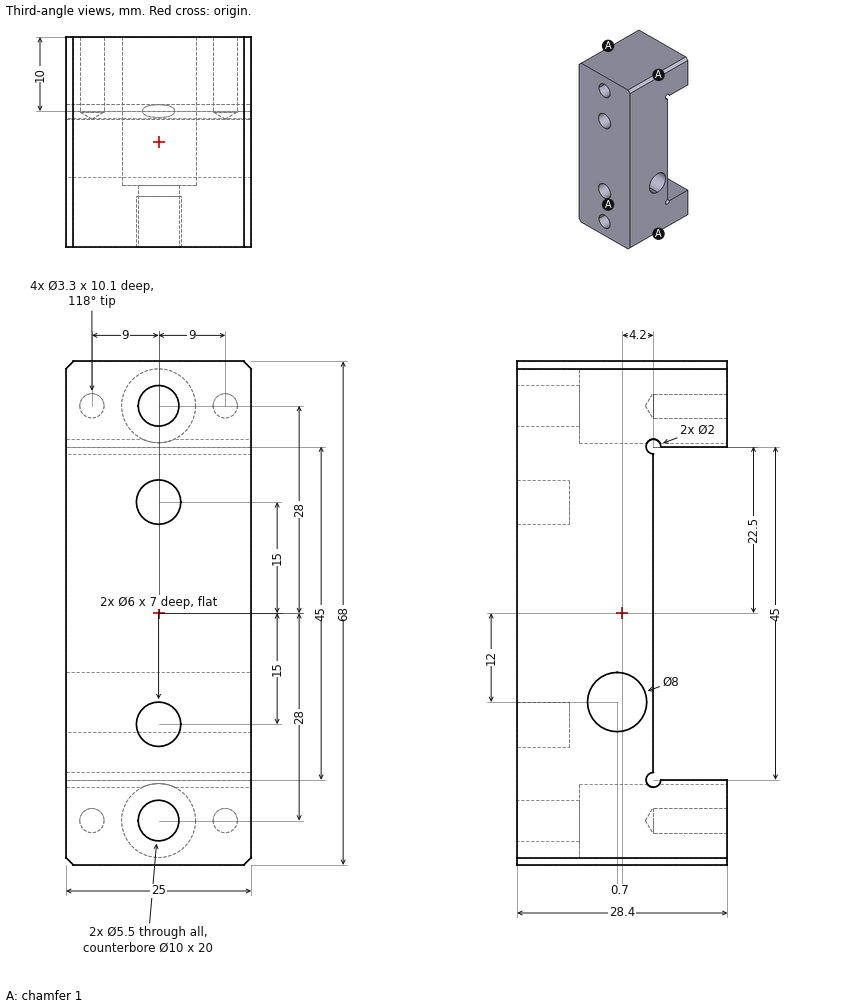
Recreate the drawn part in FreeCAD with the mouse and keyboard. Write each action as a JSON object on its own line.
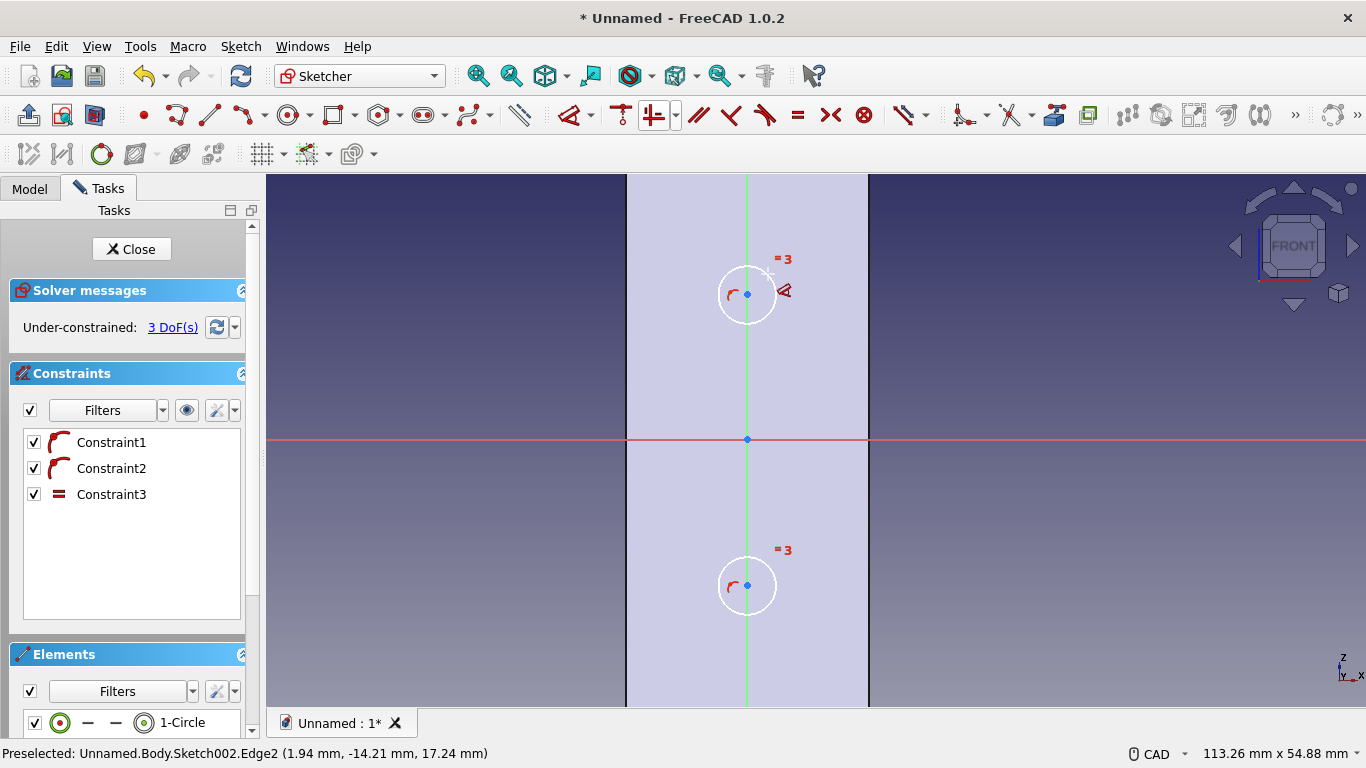
{"action": "left_click", "coordinate": [768, 566]}
{"action": "left_click", "coordinate": [791, 544]}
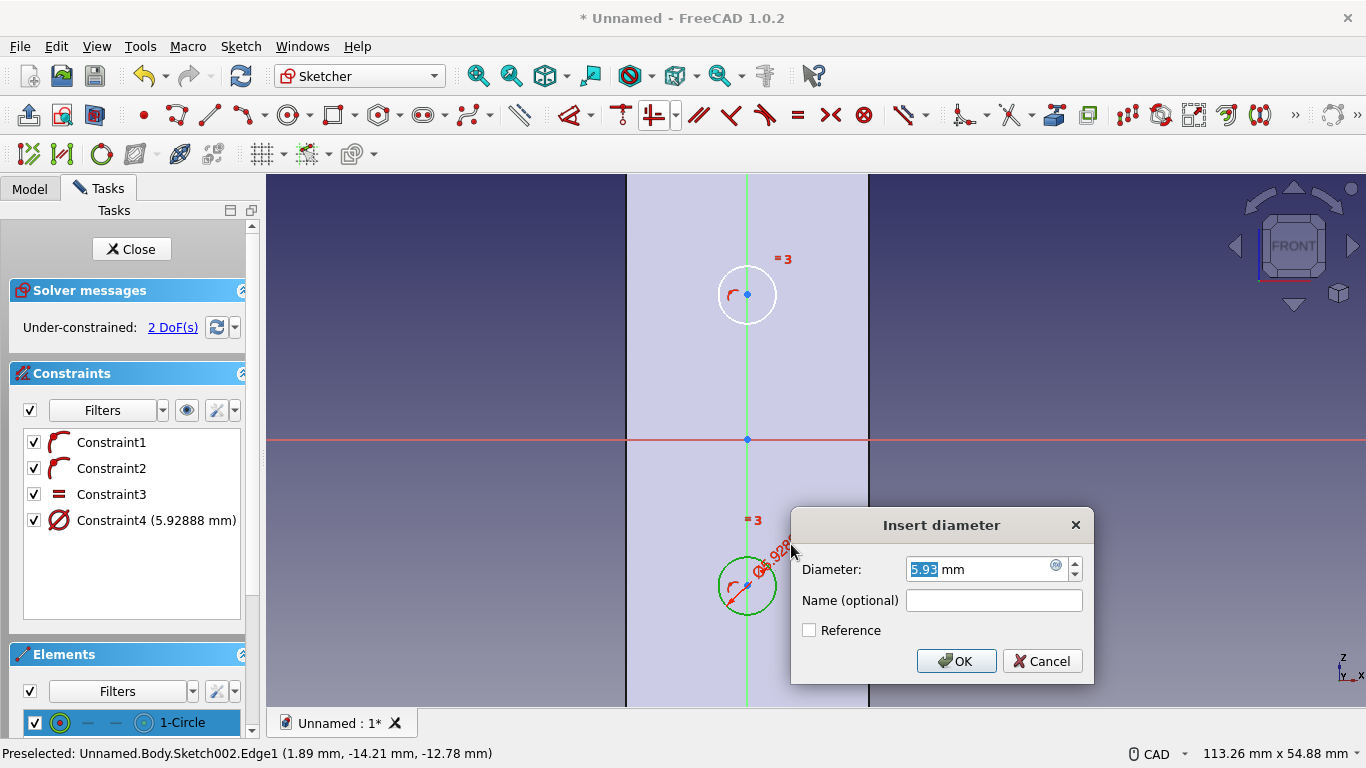
{"action": "type", "text": "6"}
{"action": "key", "text": "Return"}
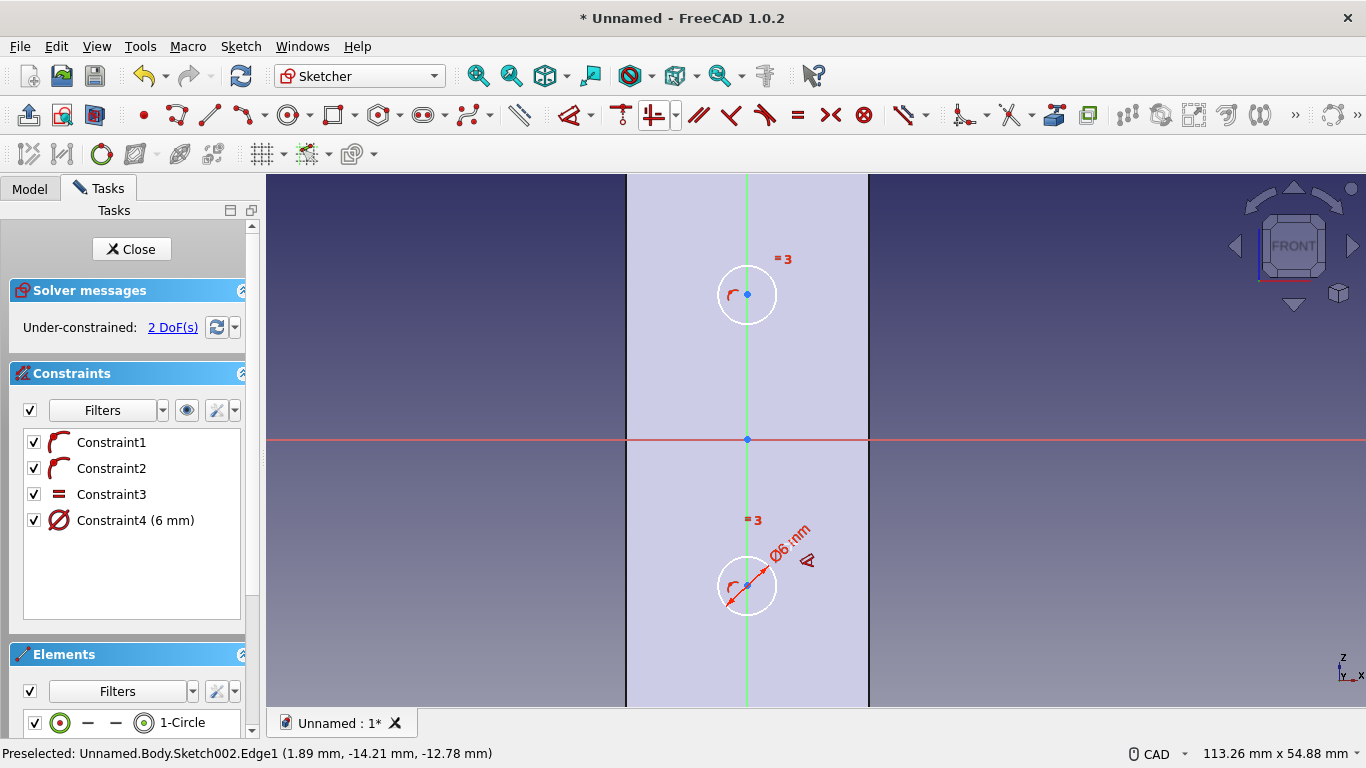
{"action": "left_click", "coordinate": [747, 586]}
{"action": "left_click", "coordinate": [781, 513]}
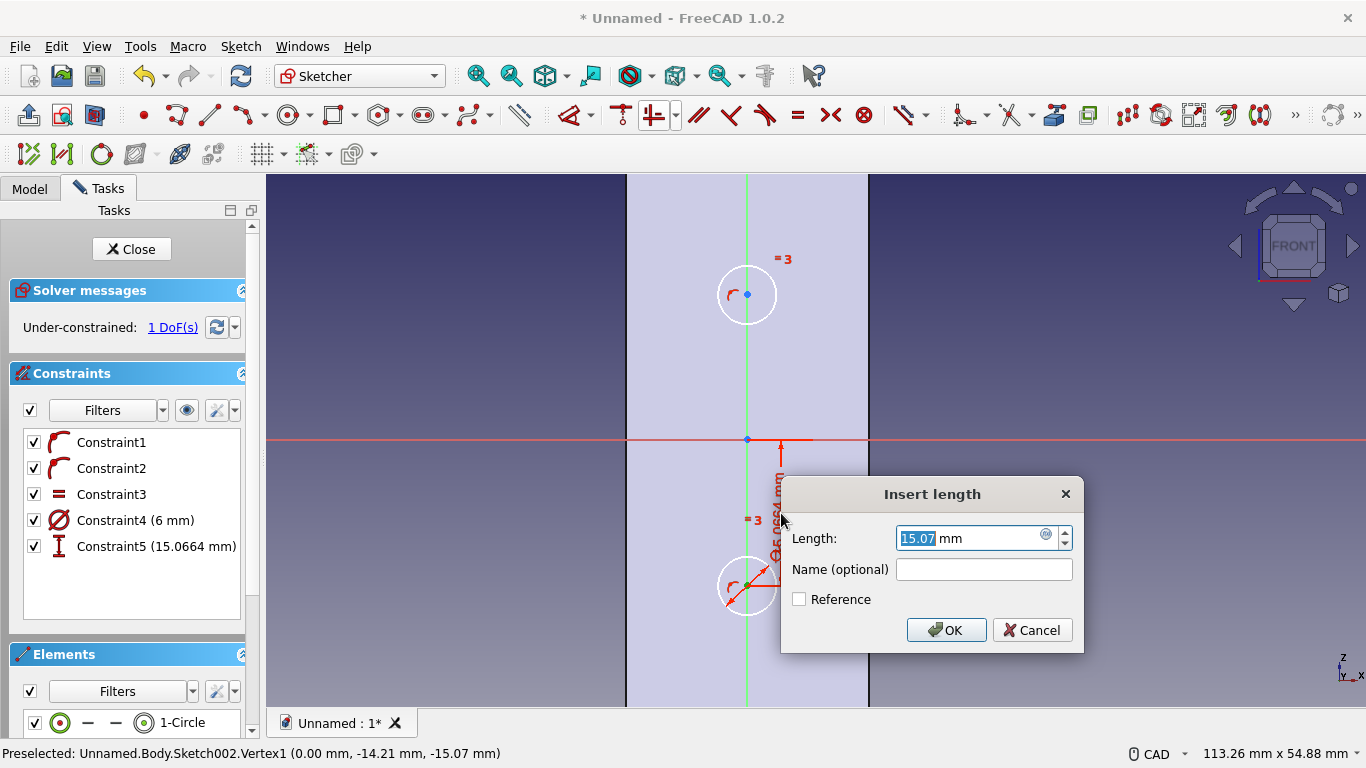
{"action": "type", "text": "15"}
{"action": "key", "text": "Return"}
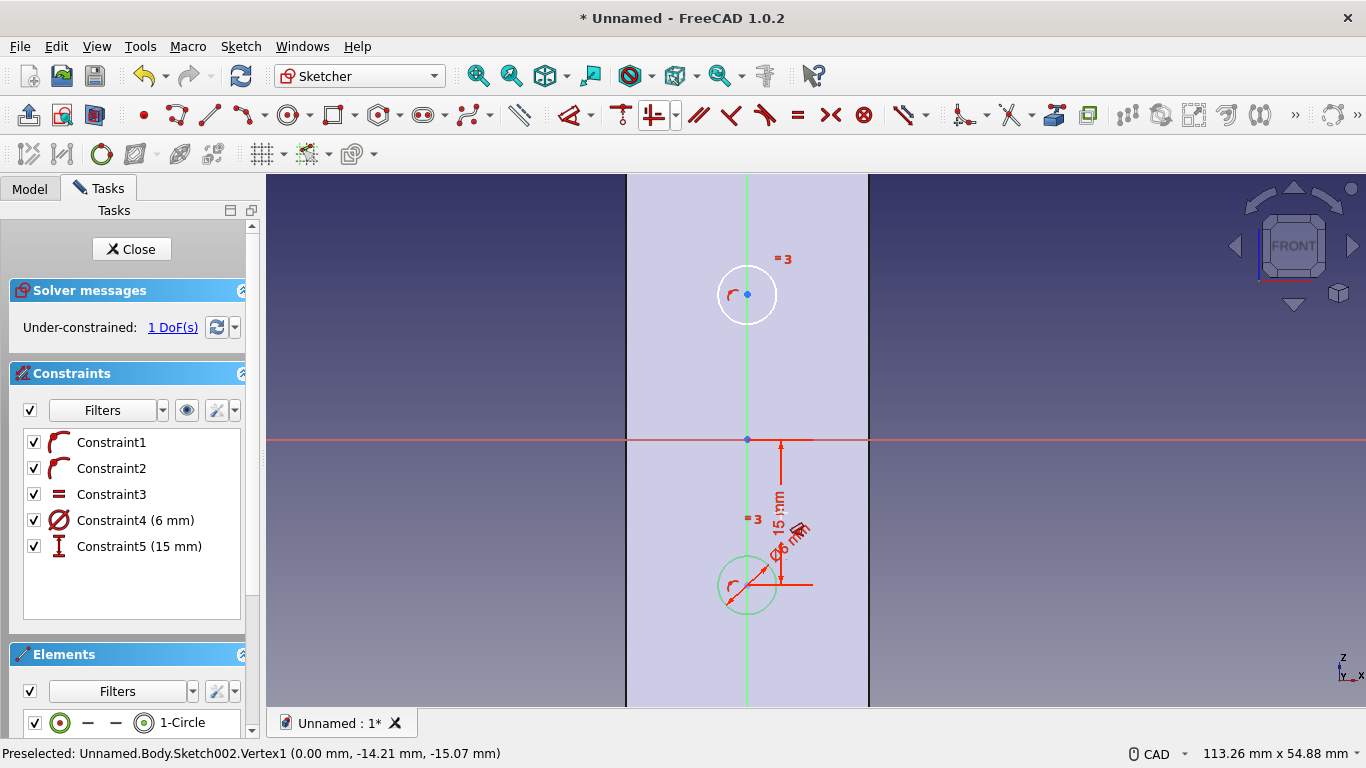
{"action": "left_click", "coordinate": [747, 295]}
{"action": "left_click", "coordinate": [781, 367]}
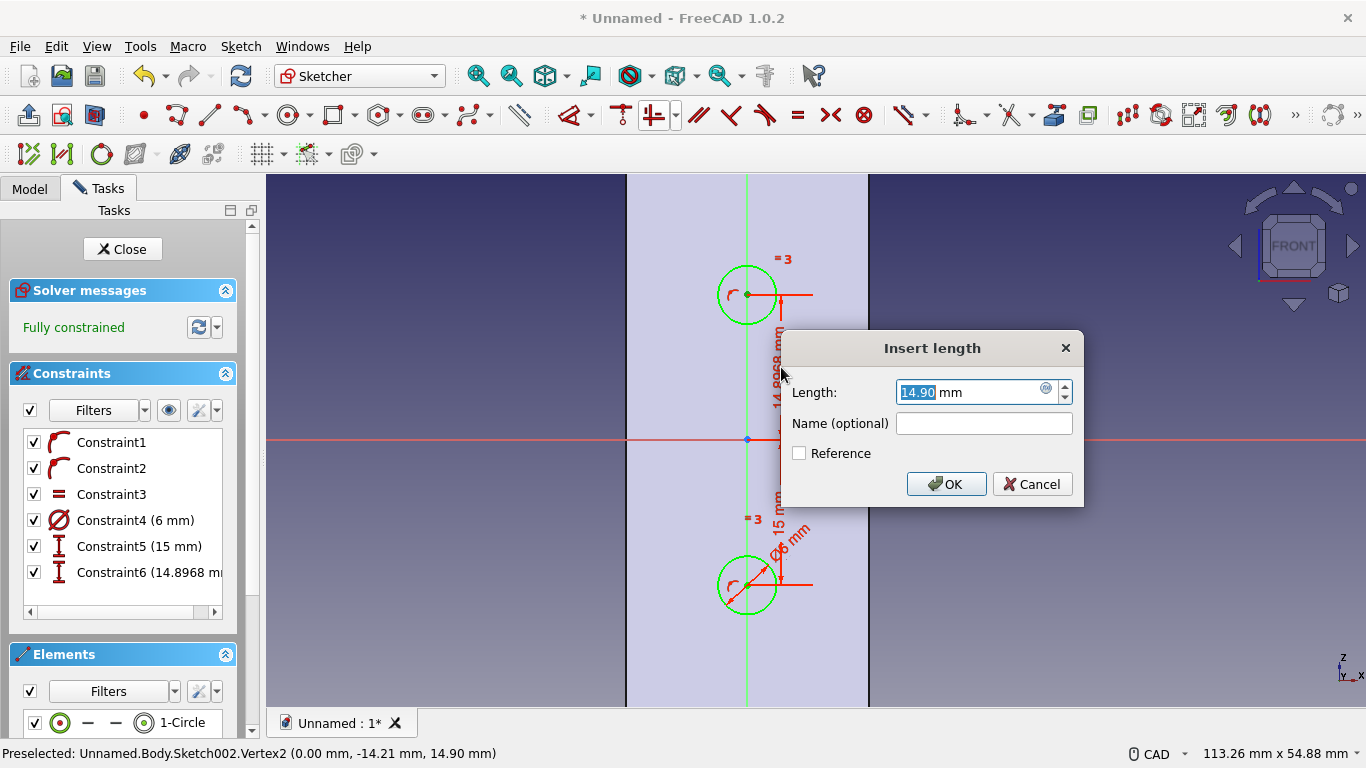
{"action": "type", "text": "15"}
{"action": "key", "text": "Return"}
{"action": "key", "text": "Escape"}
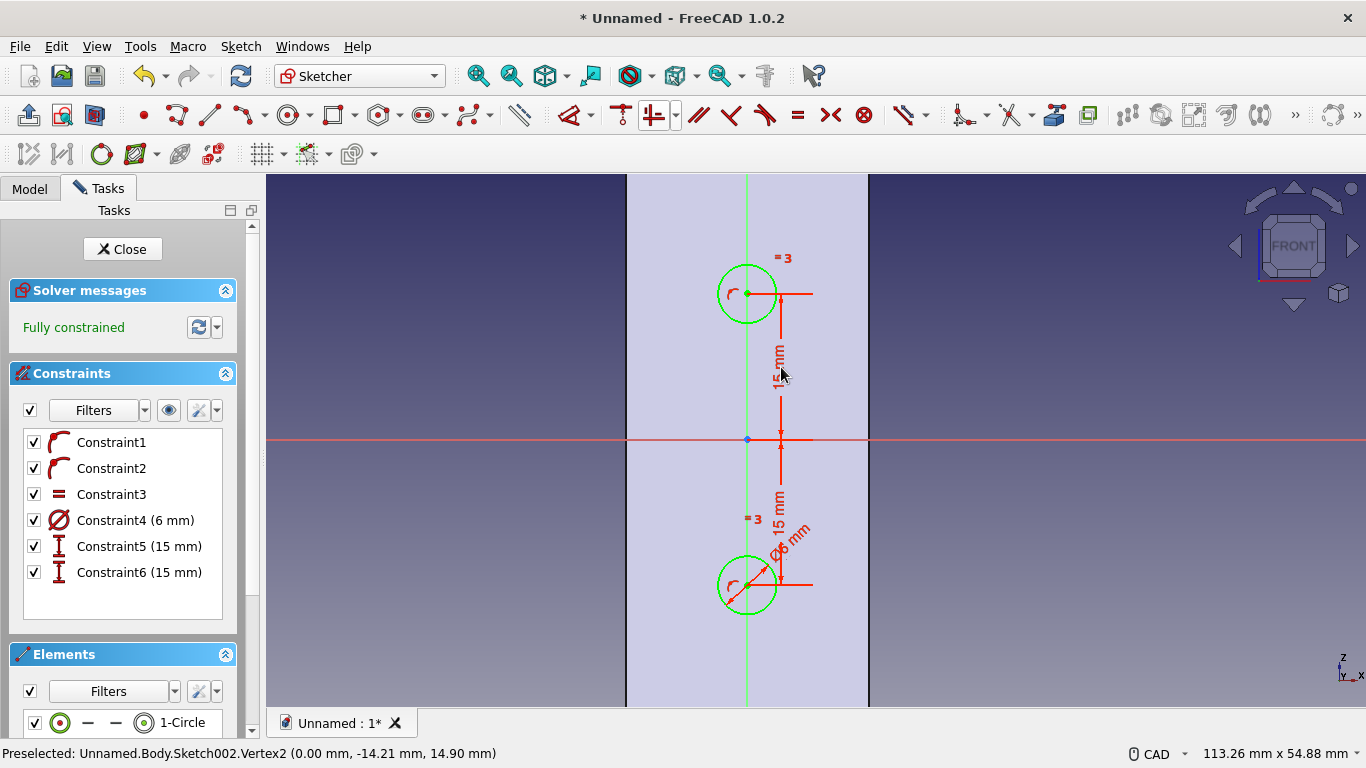
{"action": "left_click", "coordinate": [123, 249]}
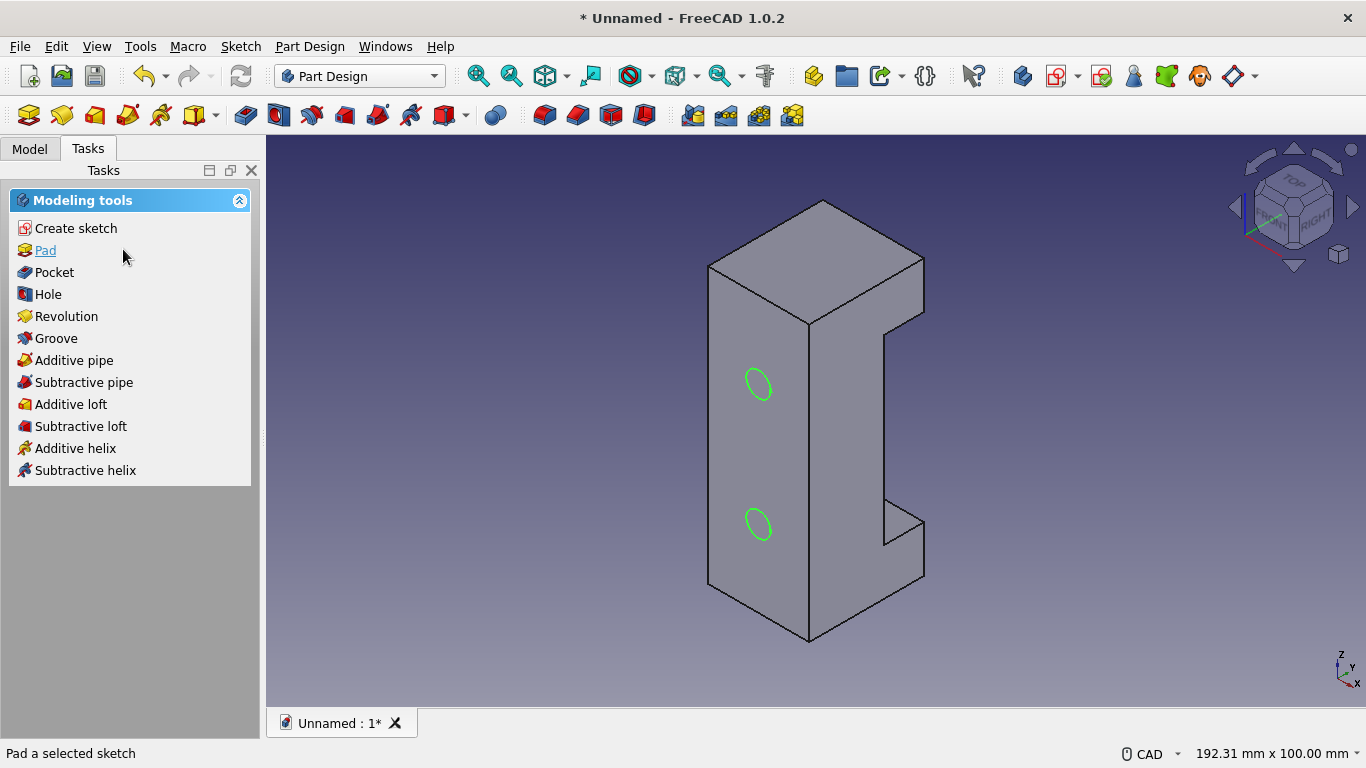
{"action": "left_click", "coordinate": [279, 116]}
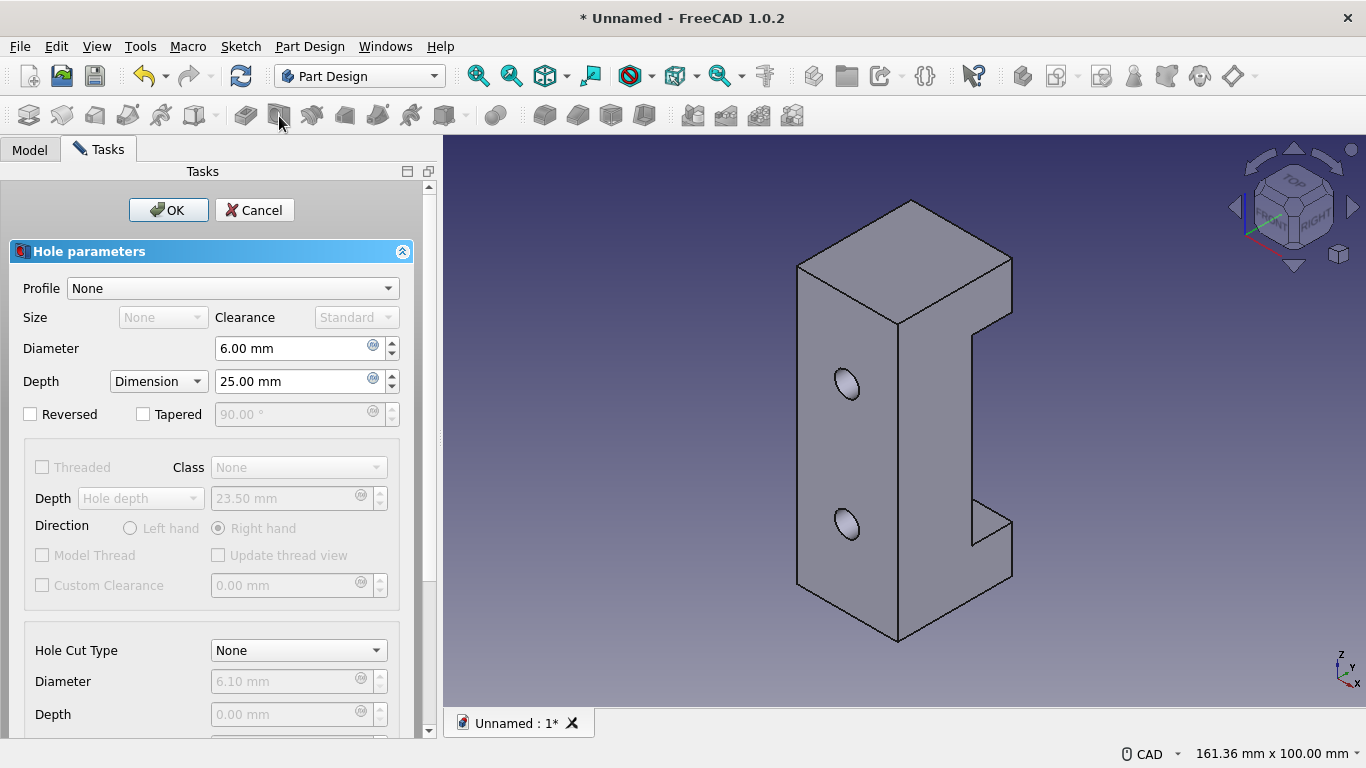
{"action": "triple_click", "coordinate": [300, 348]}